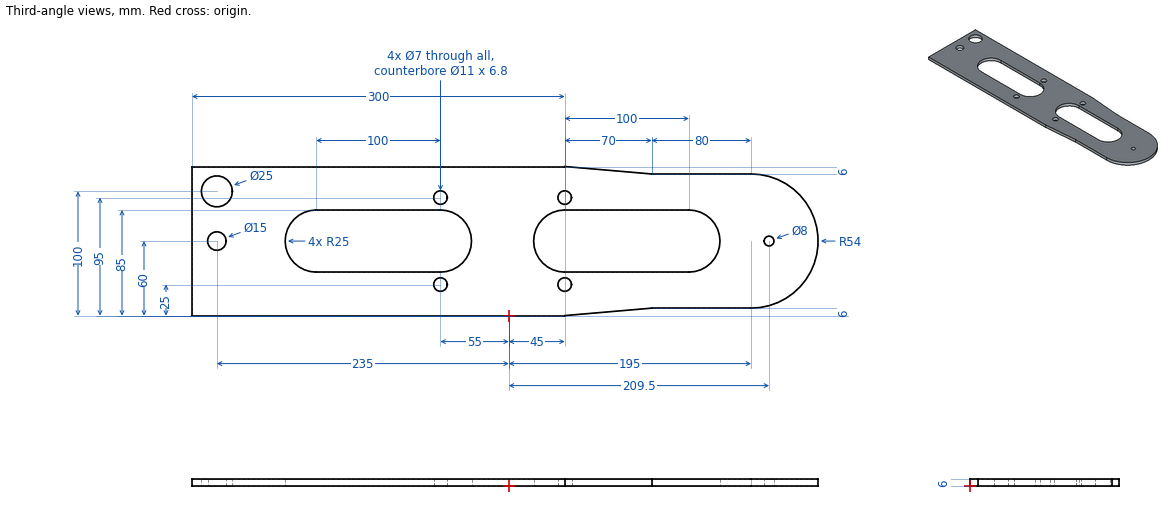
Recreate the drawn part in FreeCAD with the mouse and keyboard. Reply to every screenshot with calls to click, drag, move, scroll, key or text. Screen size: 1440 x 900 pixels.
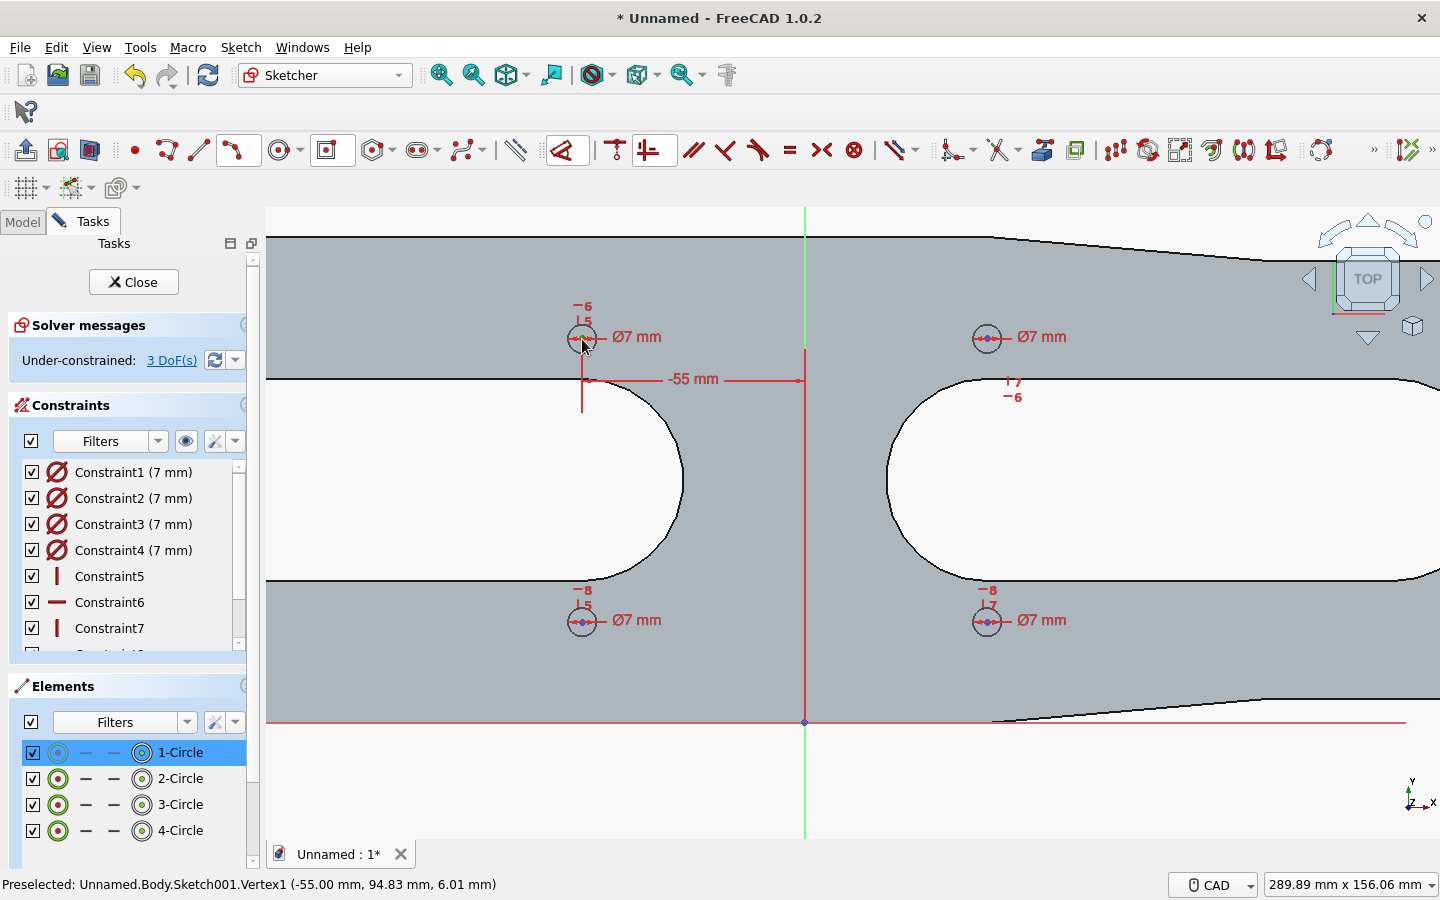
key(i)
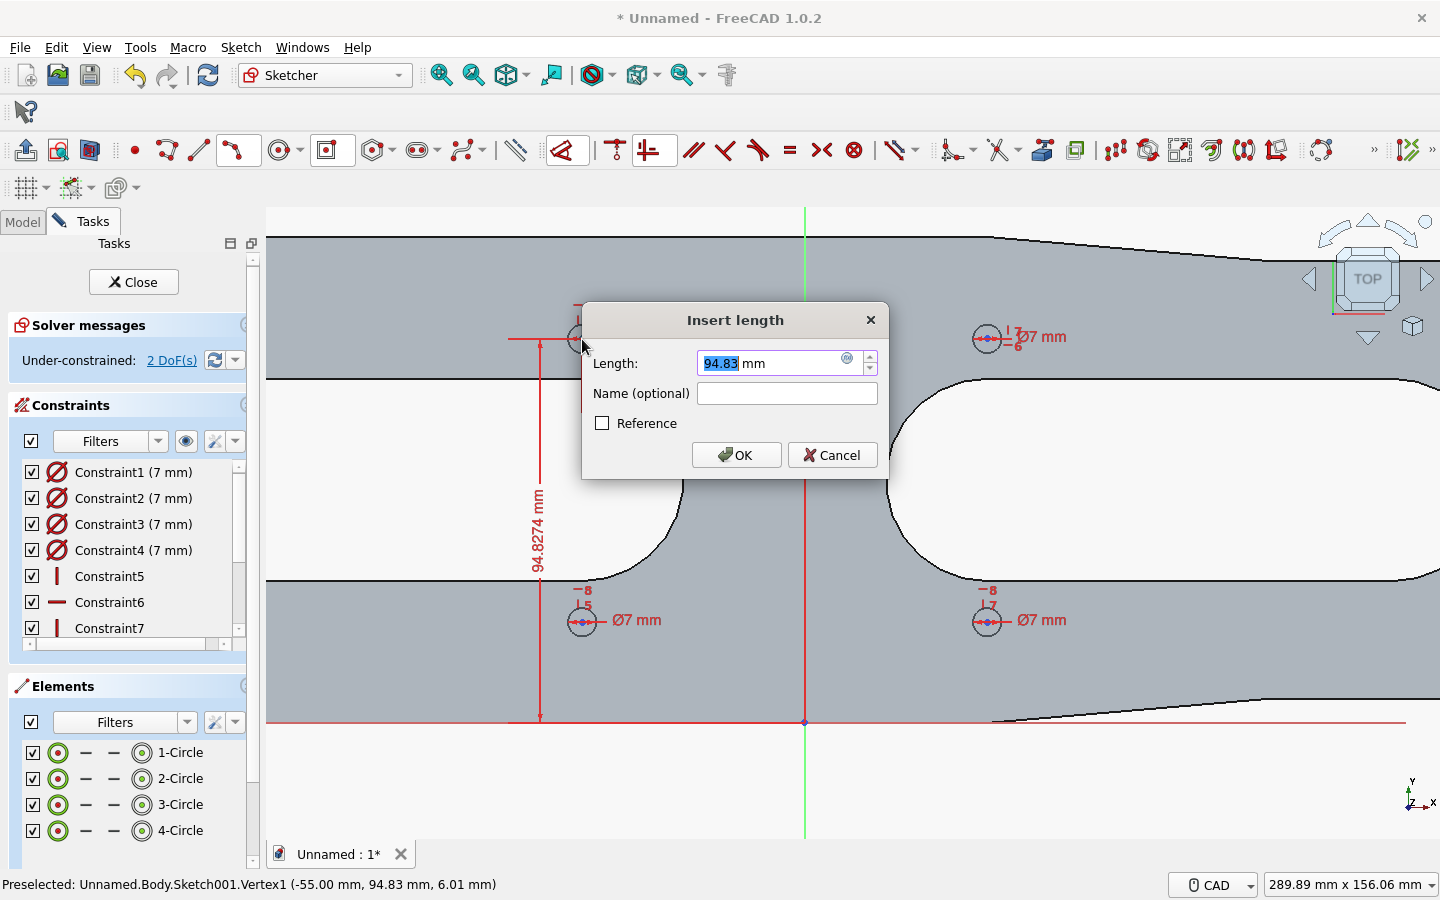
text(95)
key(Return)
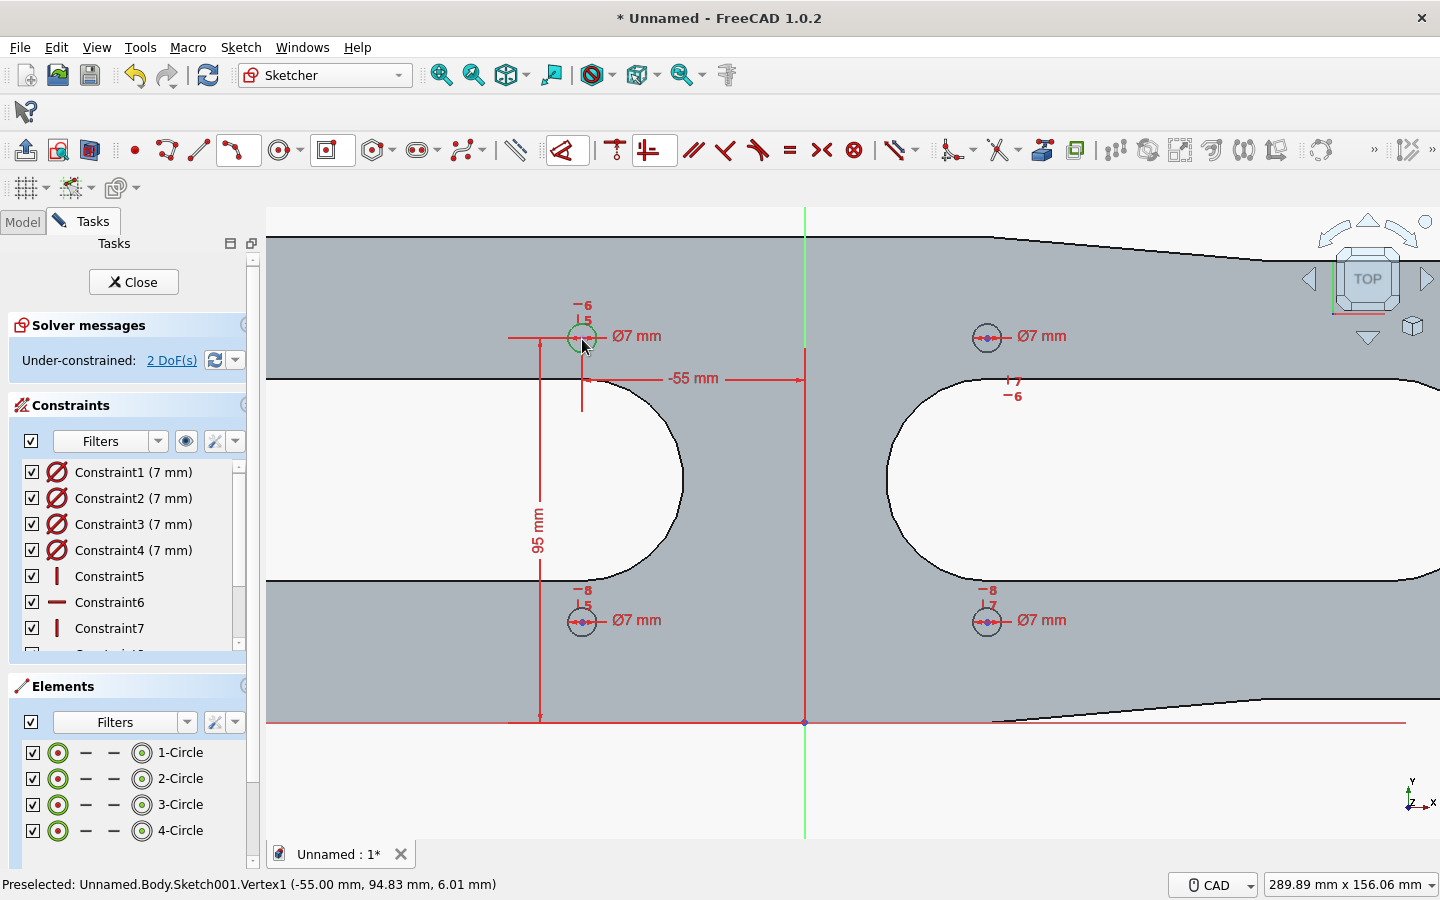
click(582, 622)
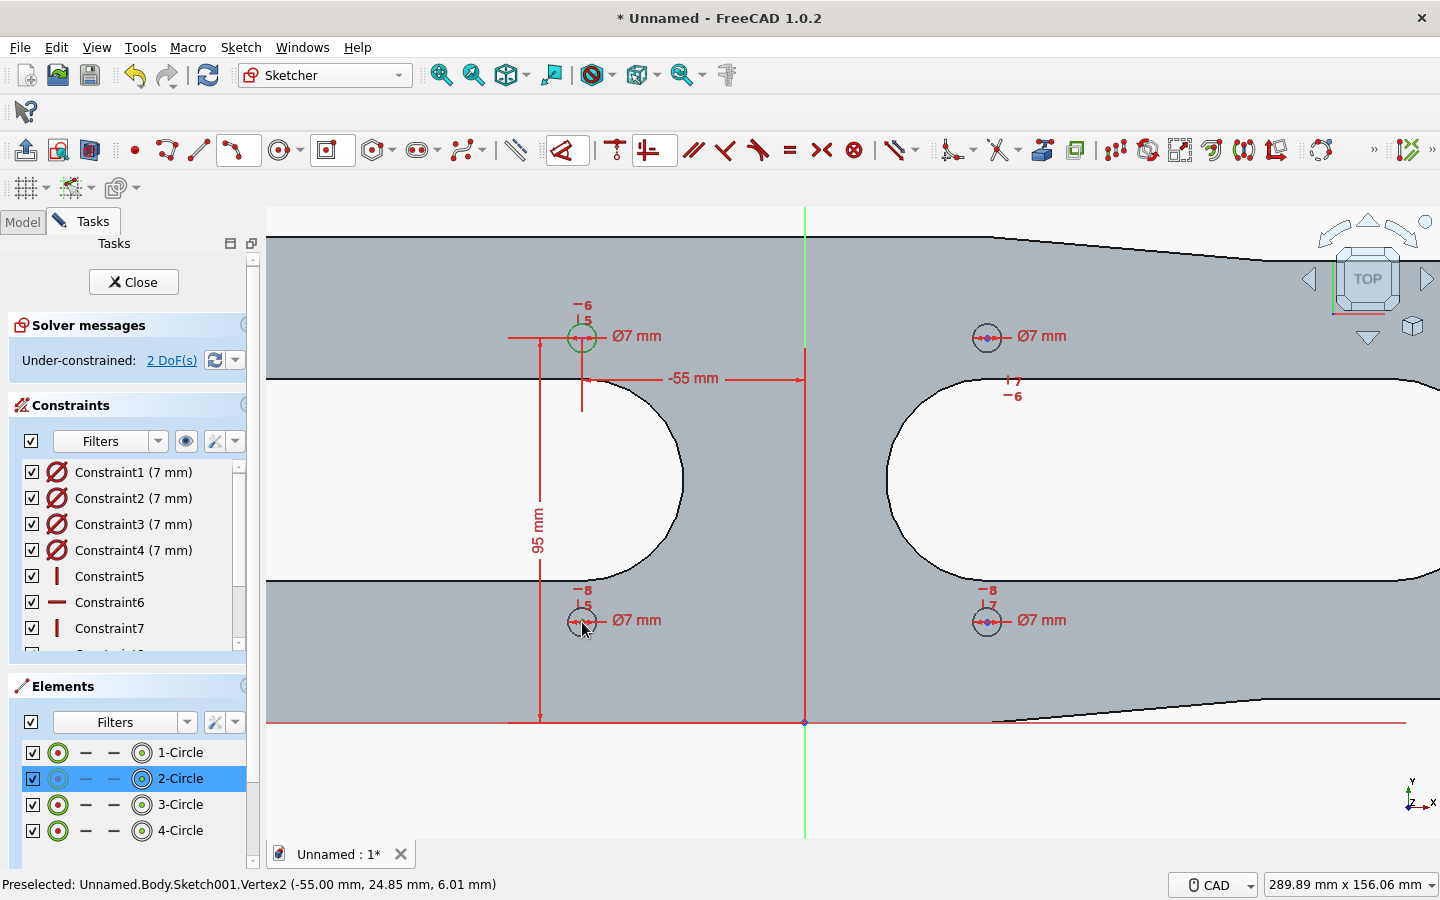
click(584, 150)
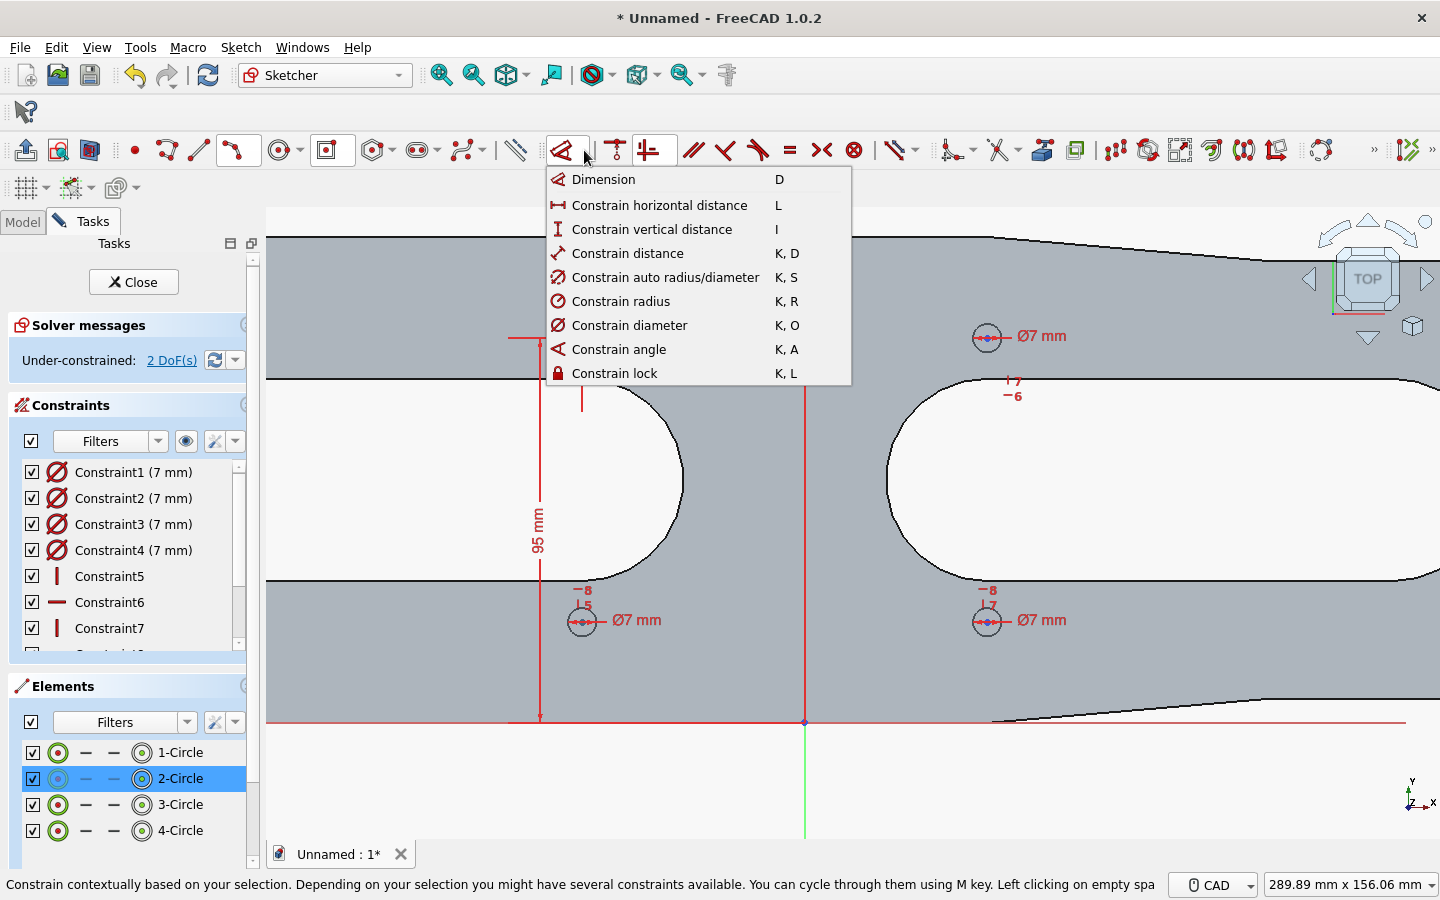
click(699, 229)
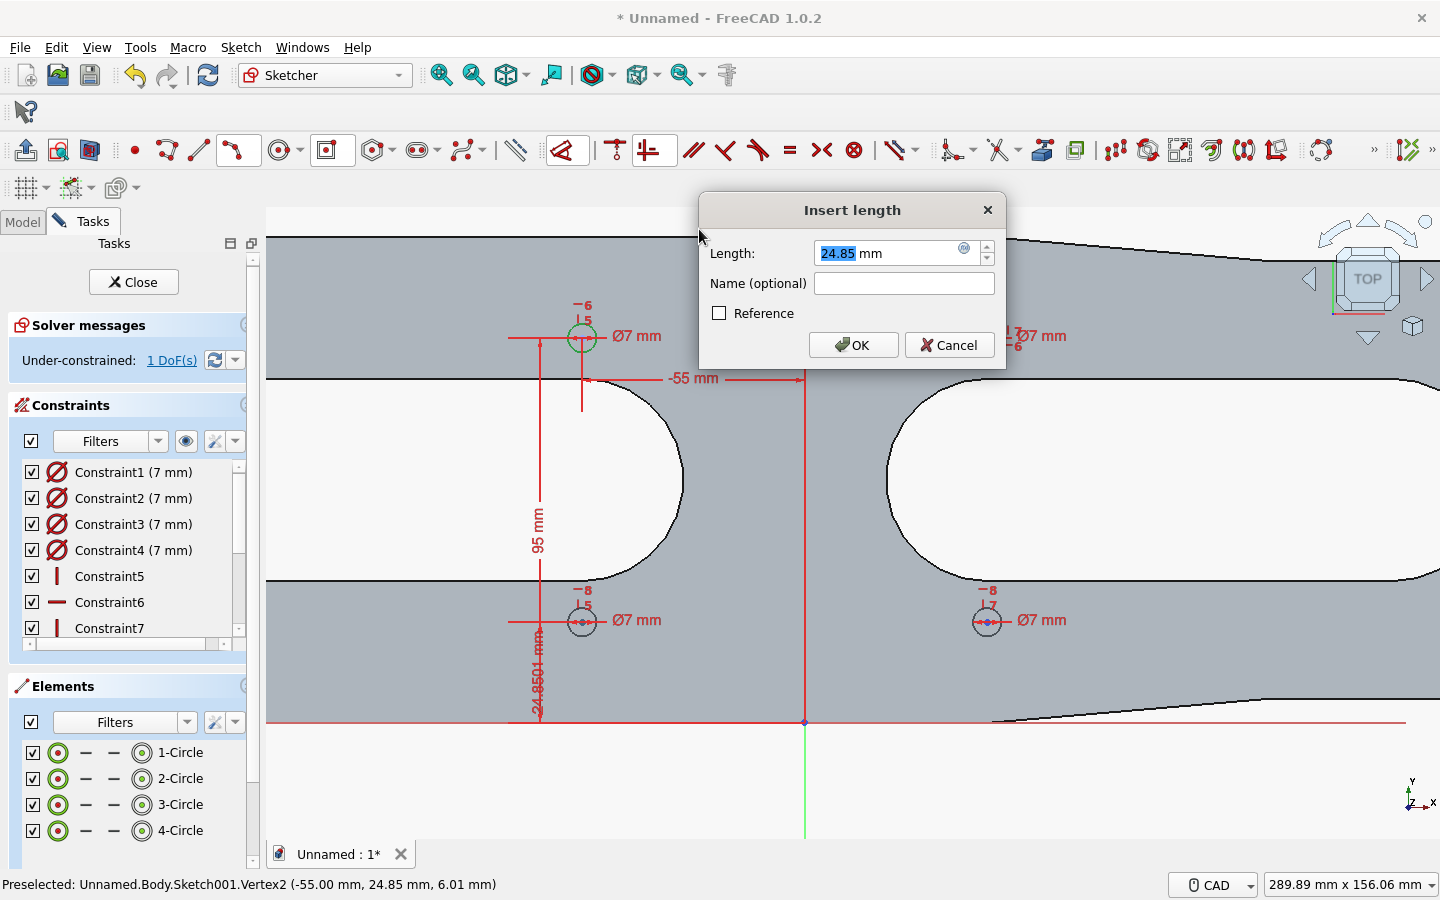
text(25)
key(Return)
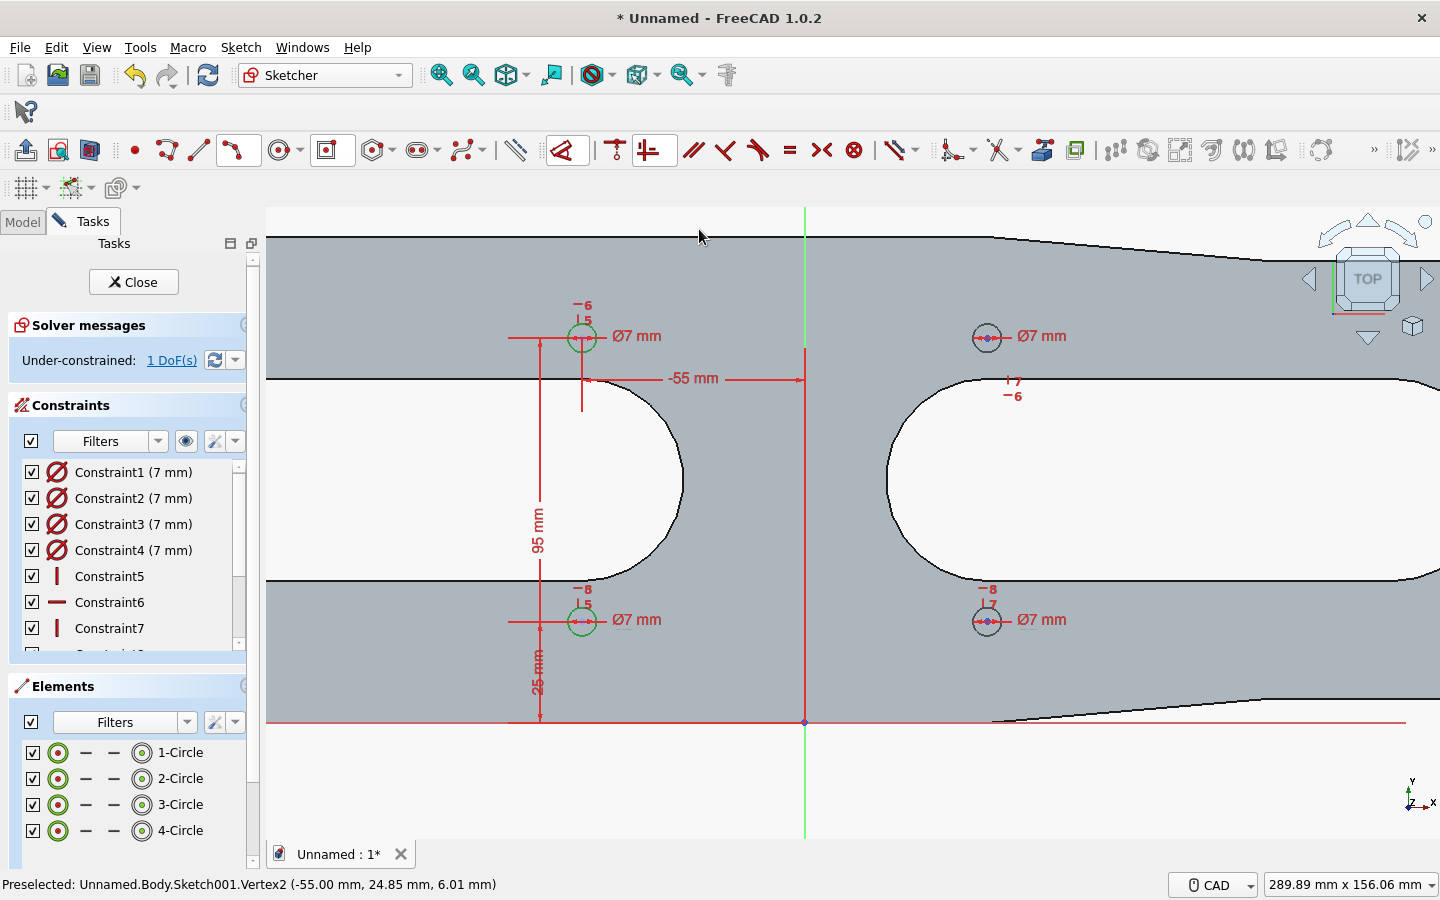
click(987, 338)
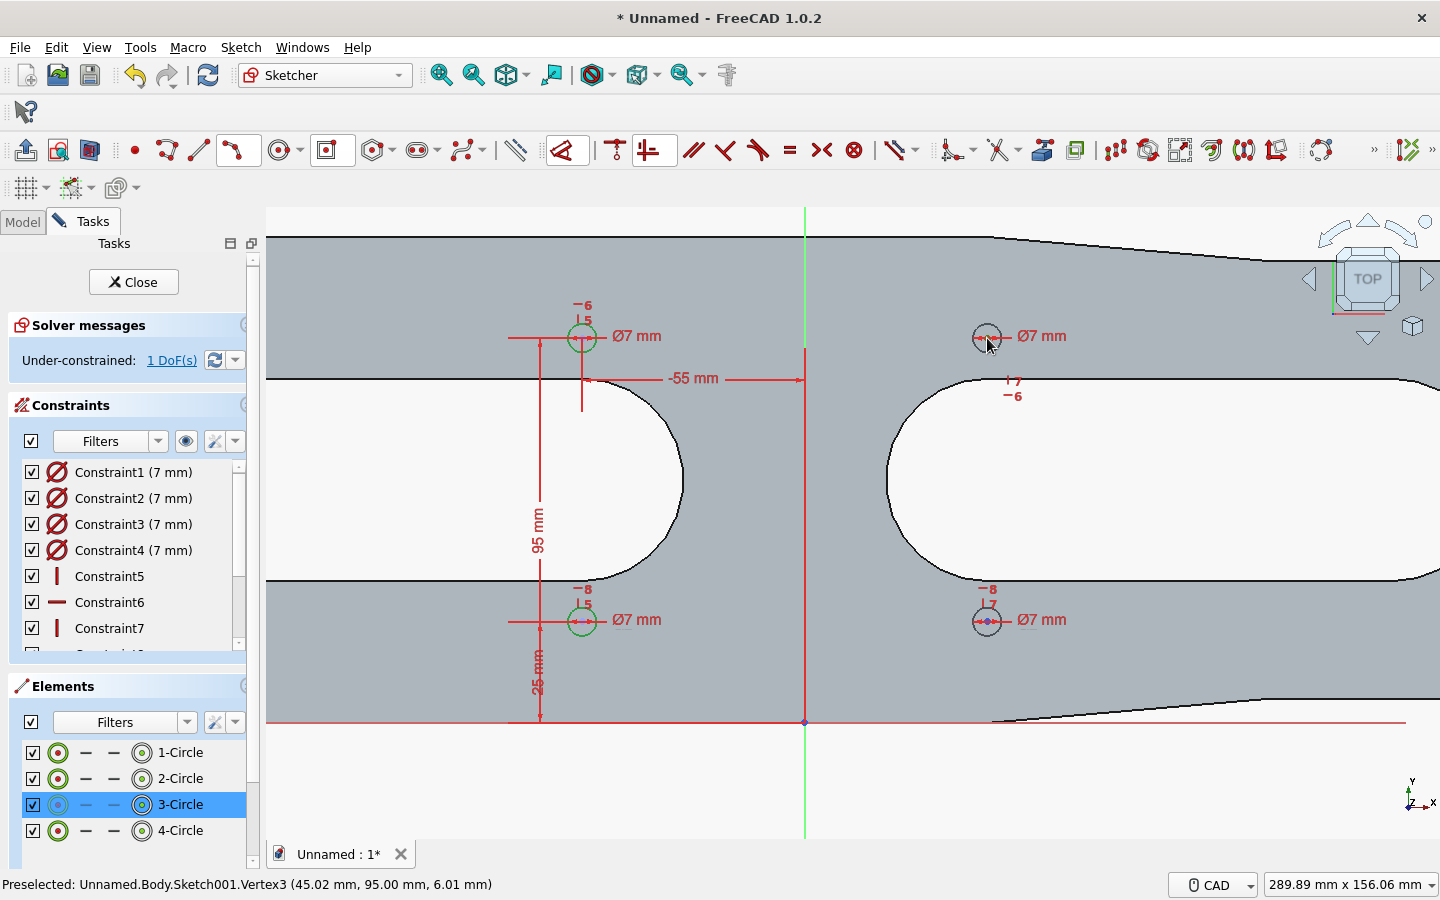
key(l)